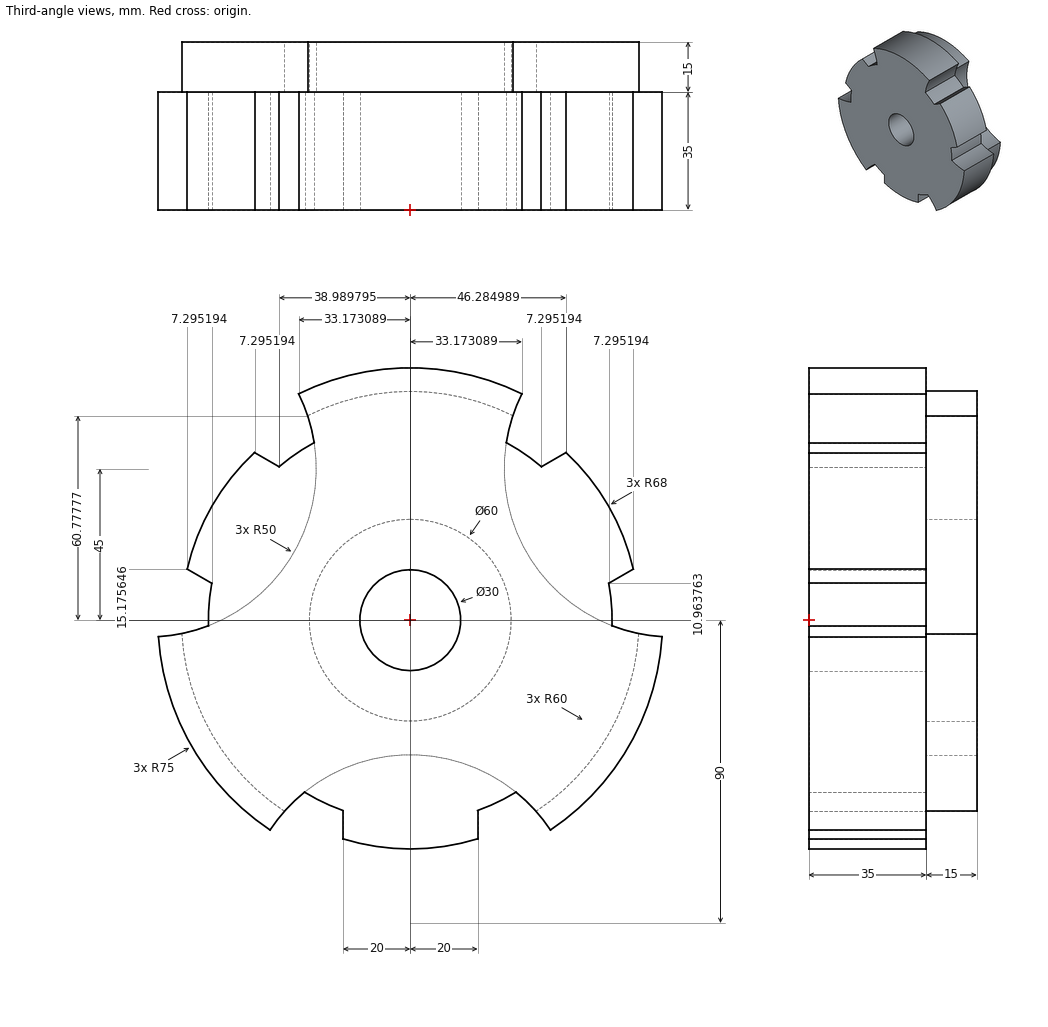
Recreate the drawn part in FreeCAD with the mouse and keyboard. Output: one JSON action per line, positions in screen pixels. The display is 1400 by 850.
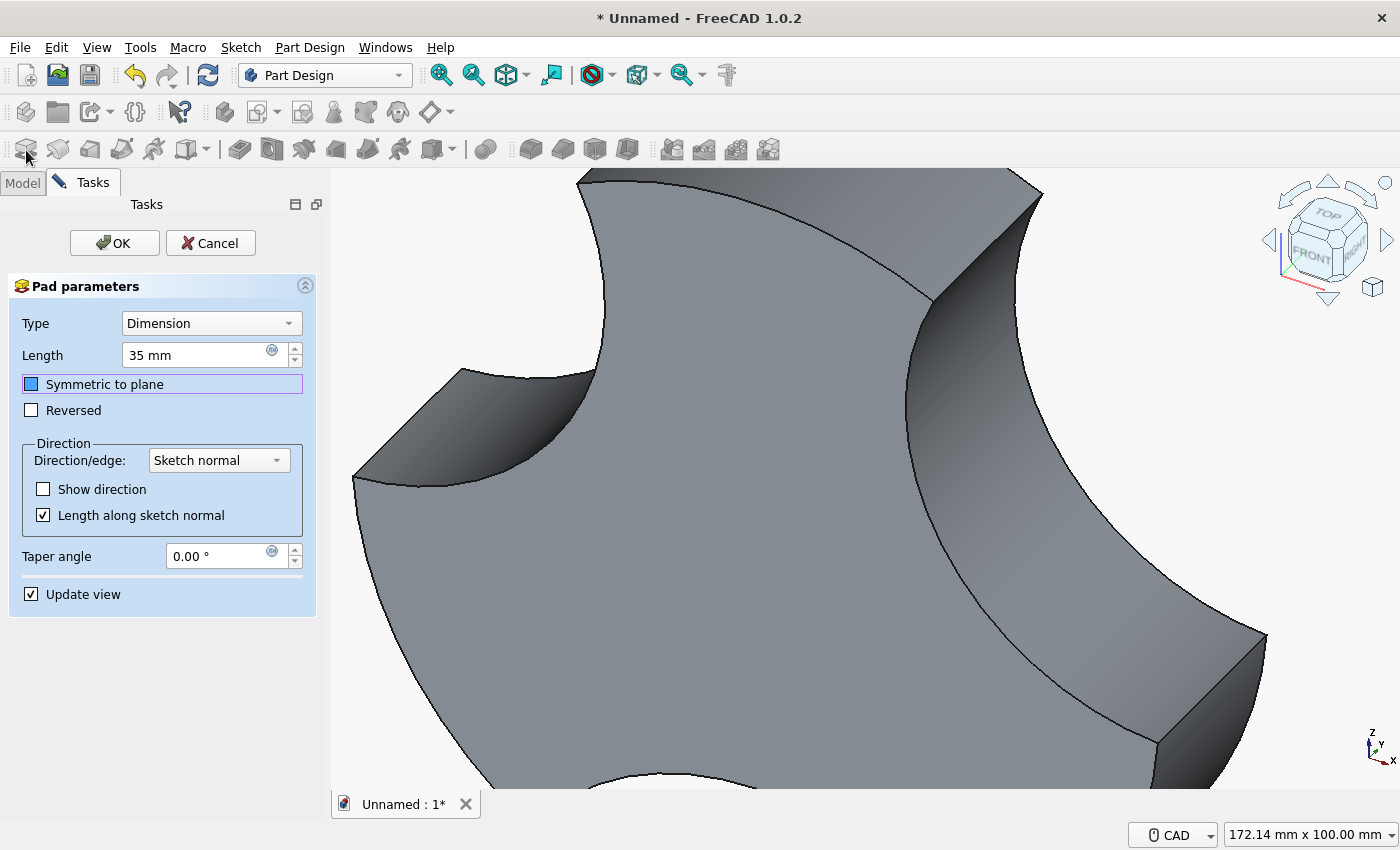
{"action": "left_click", "coordinate": [30, 410]}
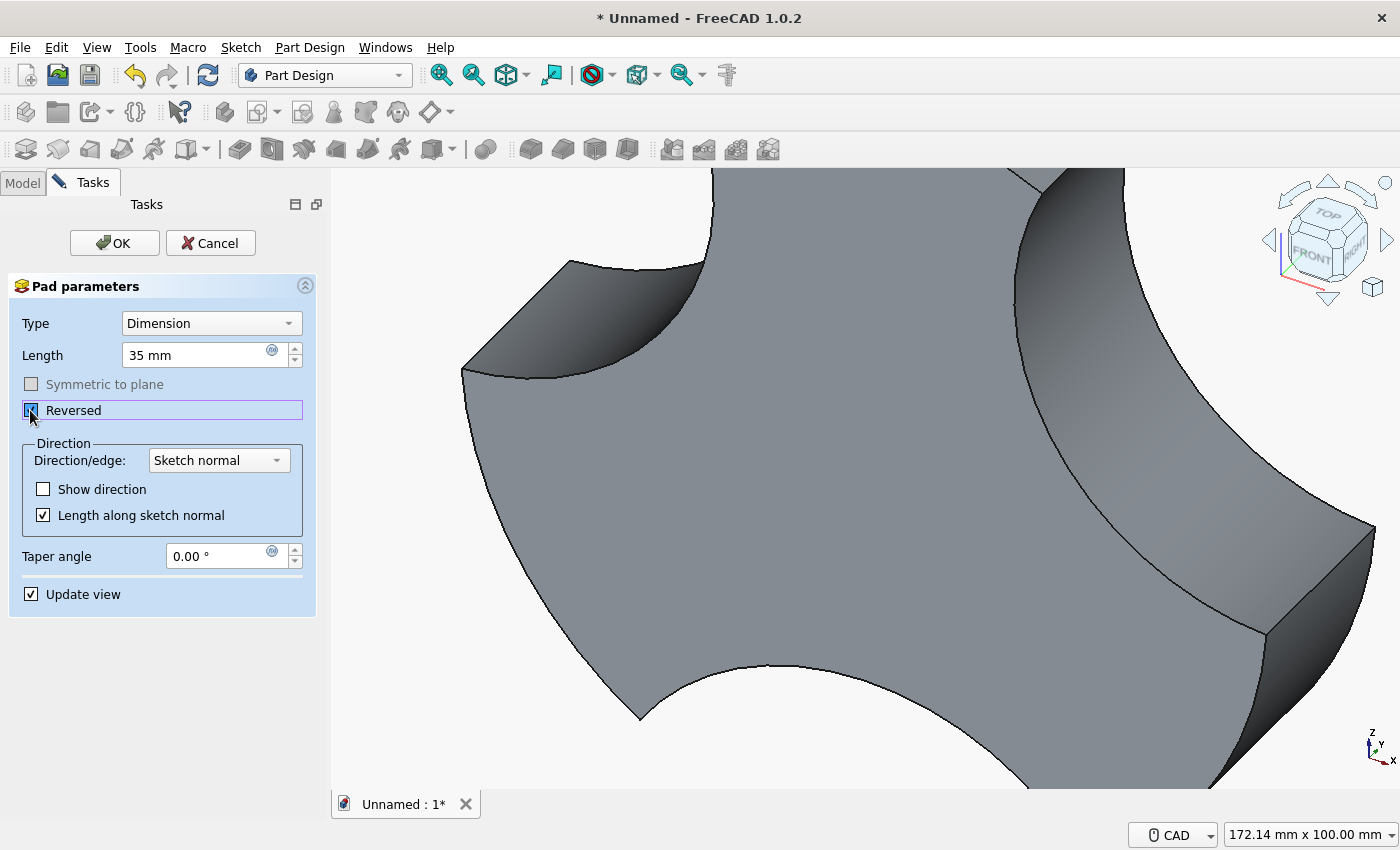
{"action": "left_click", "coordinate": [115, 243]}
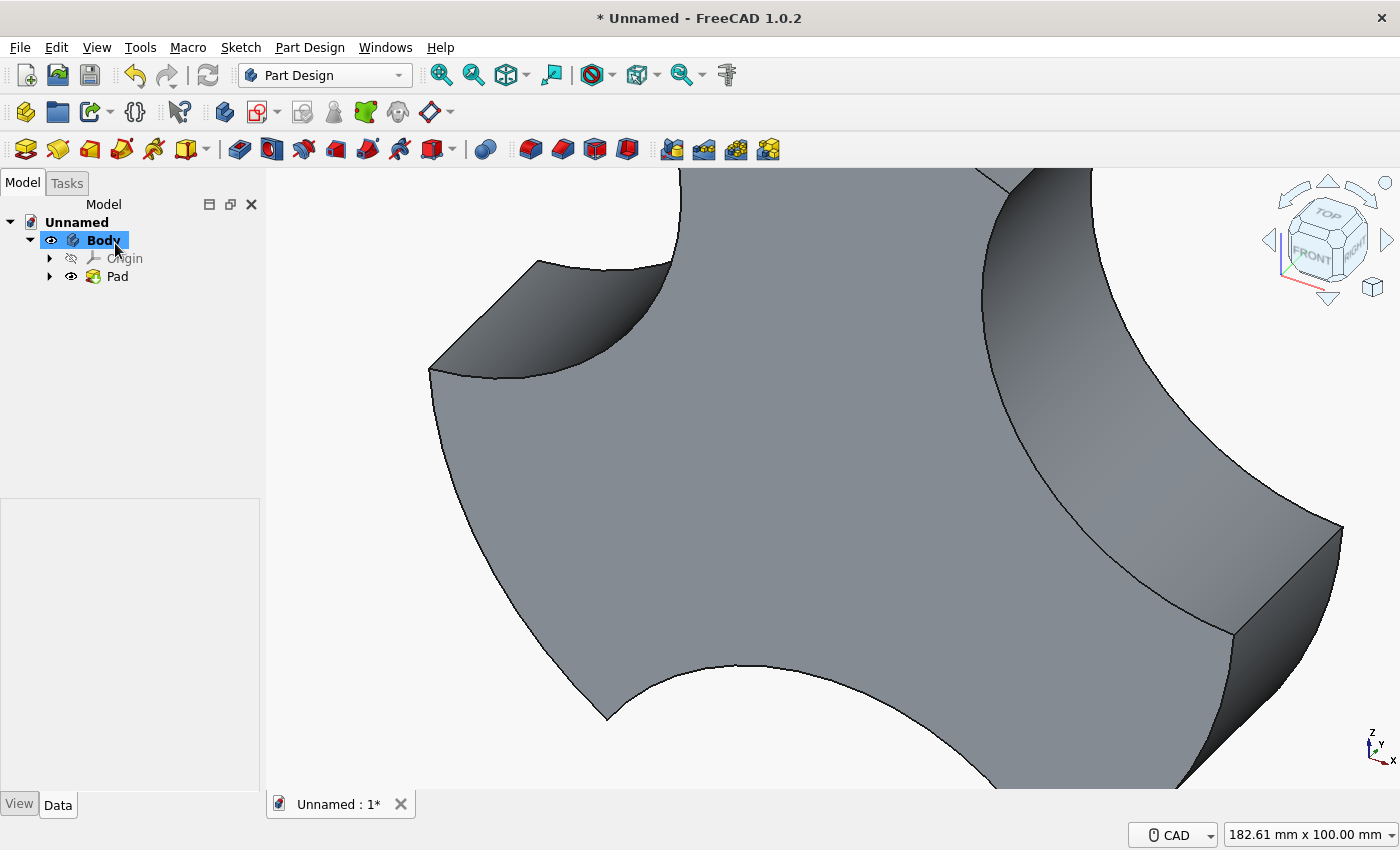
{"action": "left_click", "coordinate": [442, 76]}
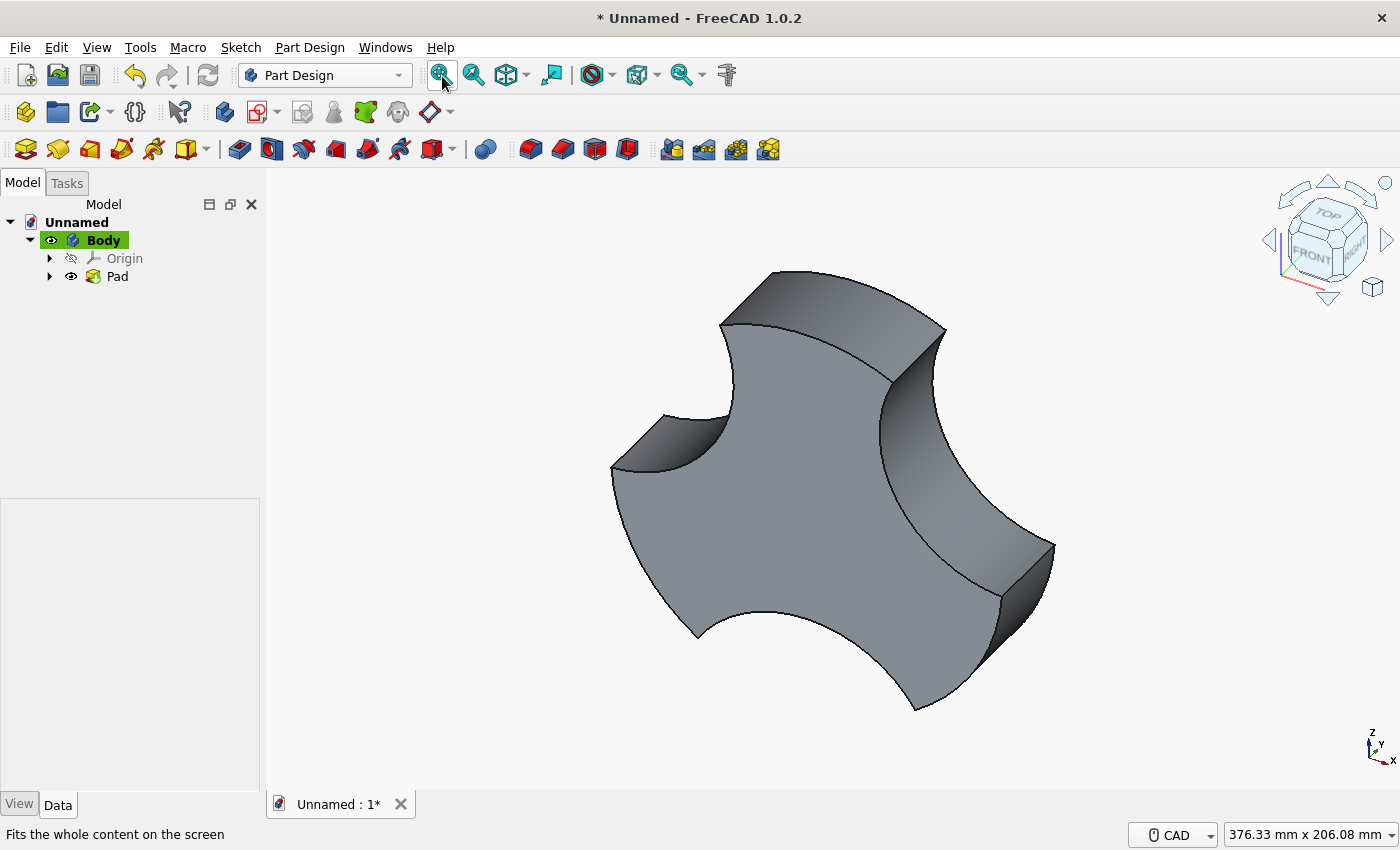
{"action": "left_click", "coordinate": [258, 112]}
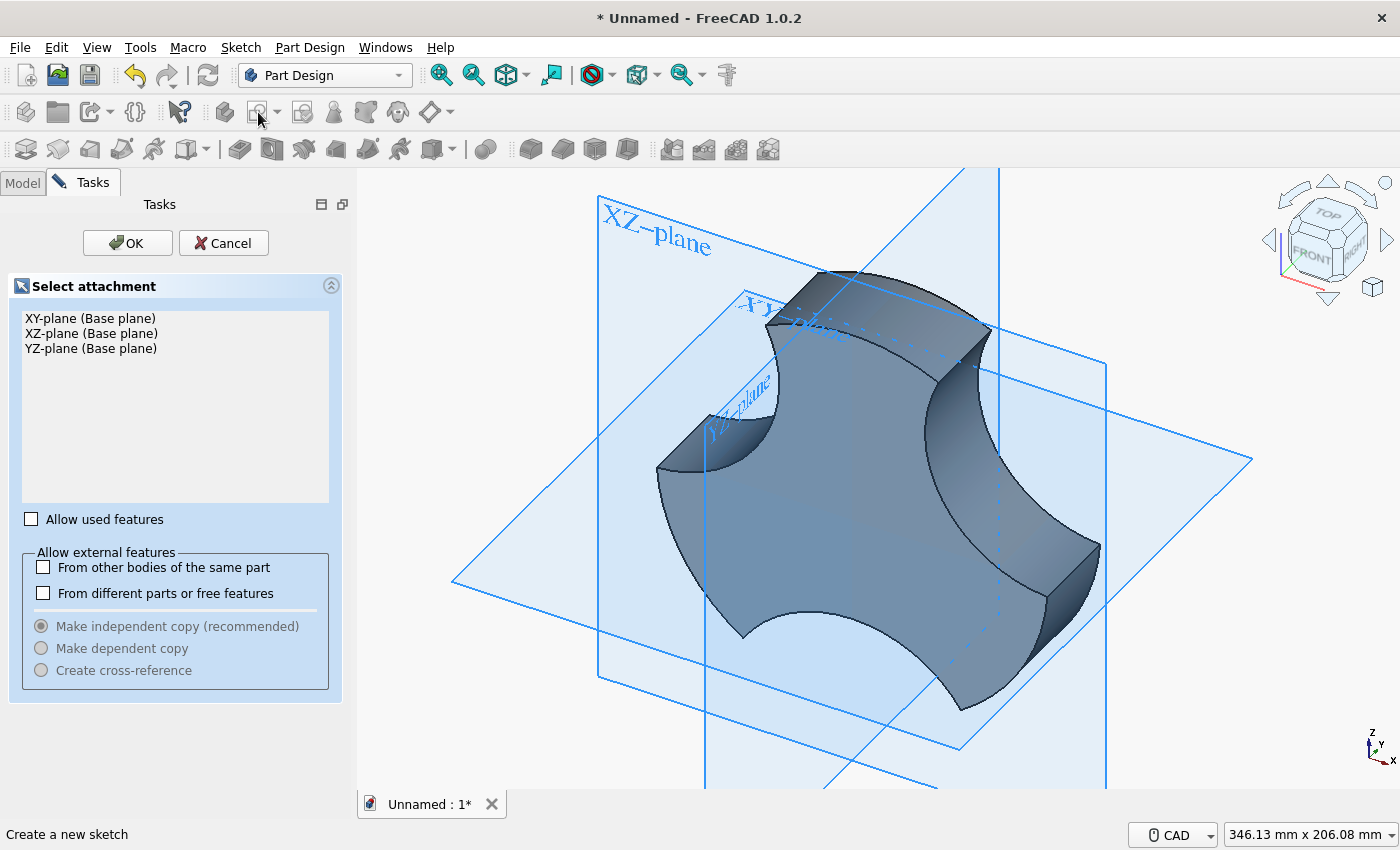
{"action": "left_click", "coordinate": [82, 334]}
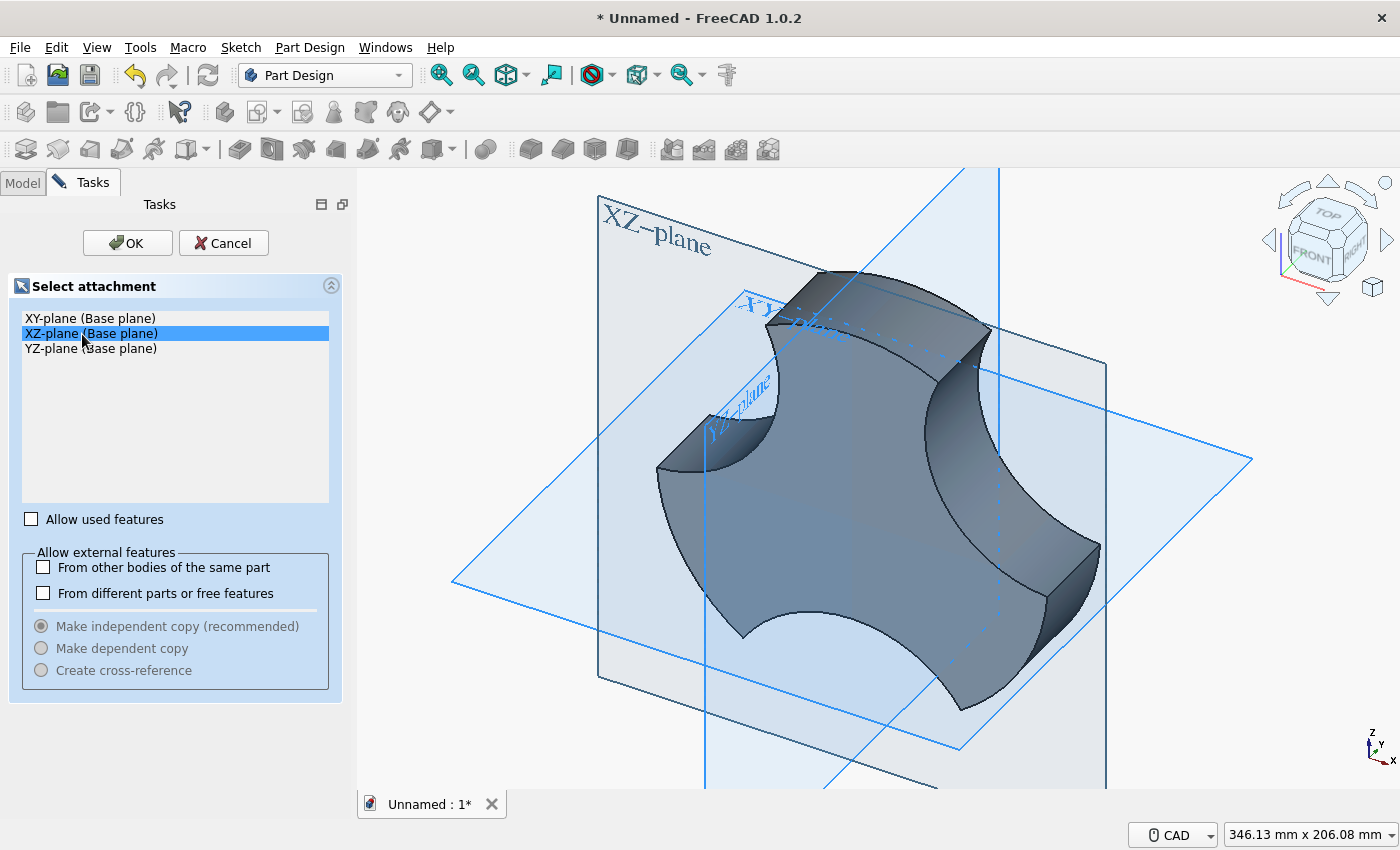
{"action": "left_click", "coordinate": [128, 243]}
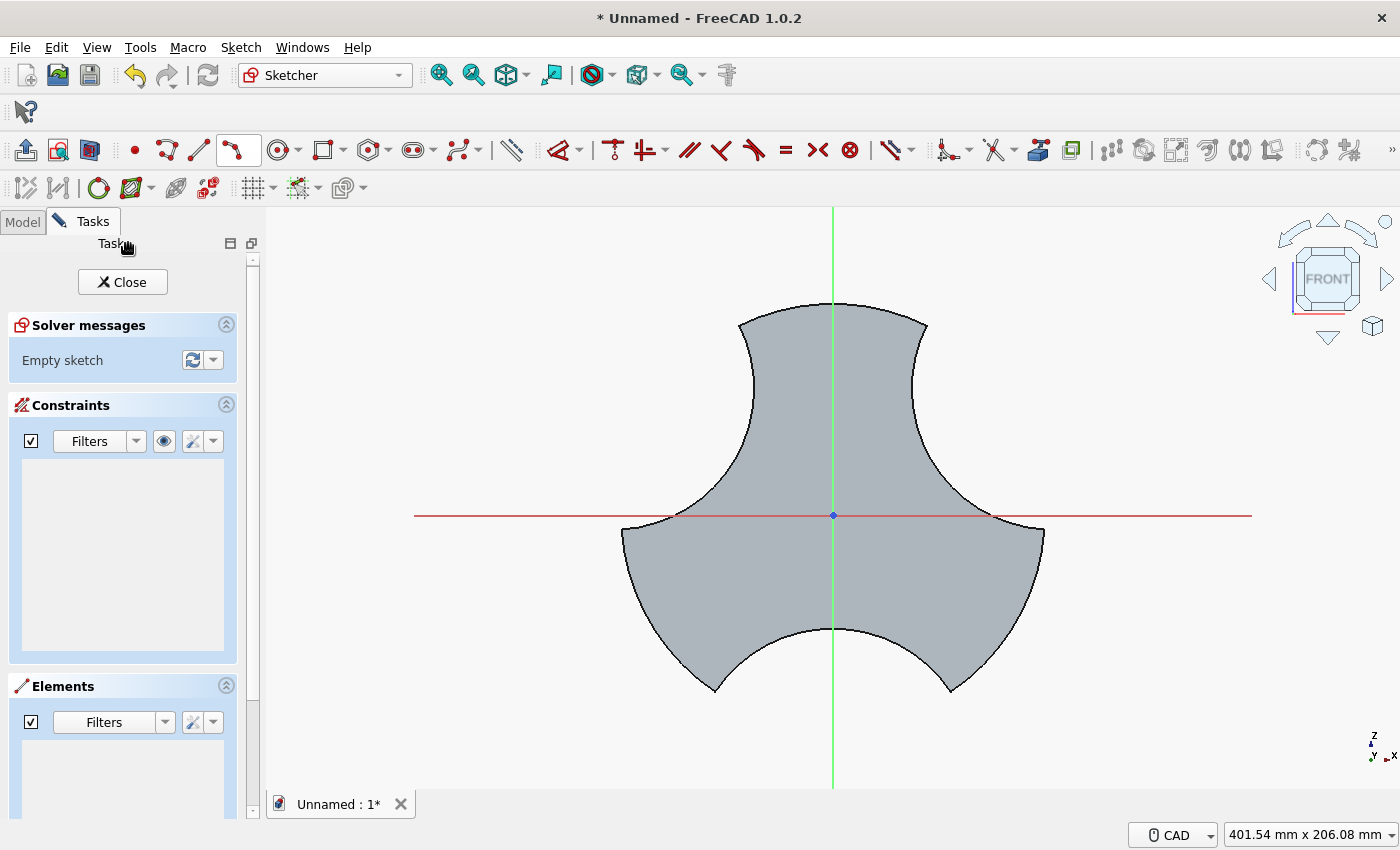
{"action": "left_click", "coordinate": [200, 150]}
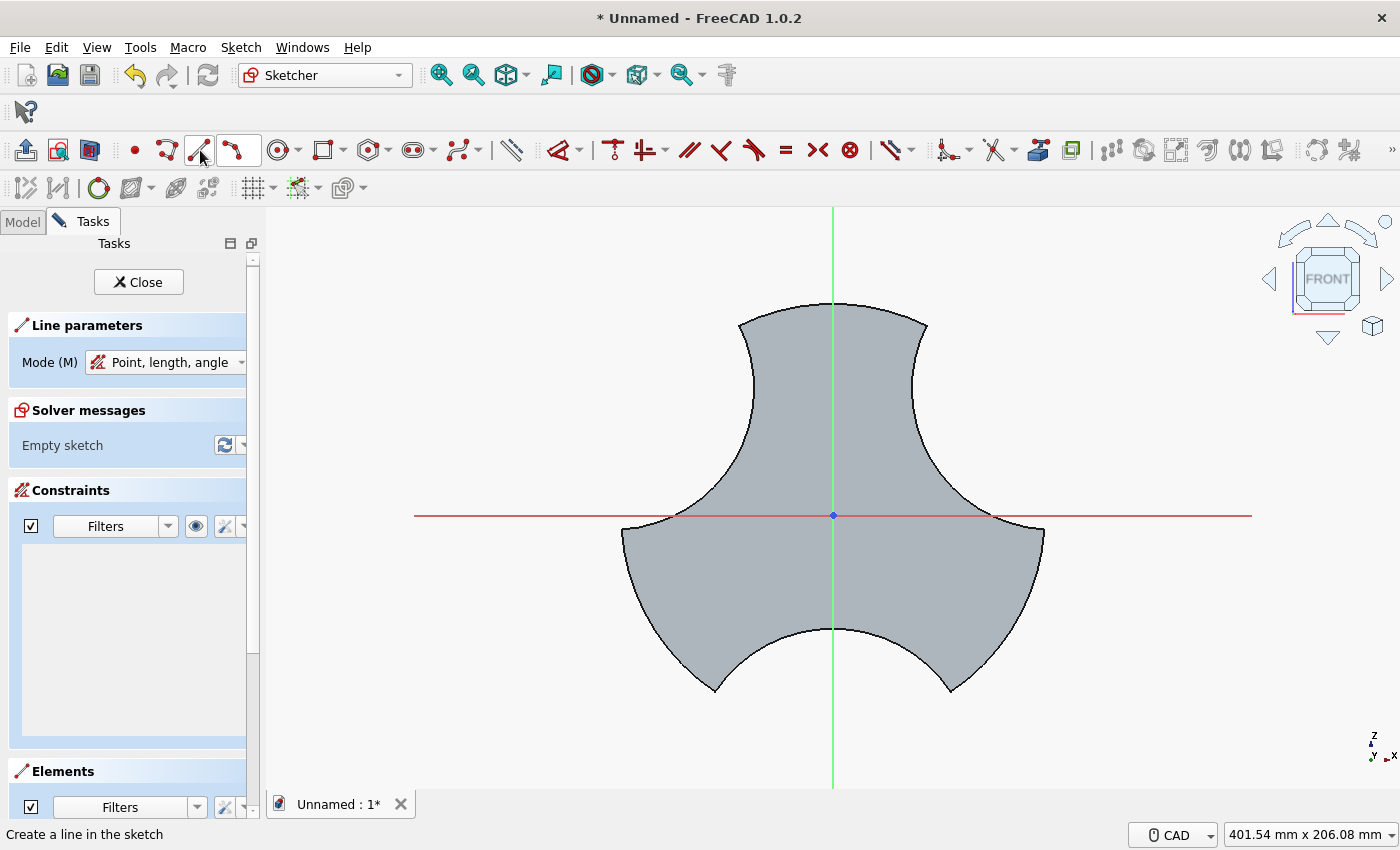
{"action": "left_click", "coordinate": [889, 699]}
{"action": "left_click", "coordinate": [889, 675]}